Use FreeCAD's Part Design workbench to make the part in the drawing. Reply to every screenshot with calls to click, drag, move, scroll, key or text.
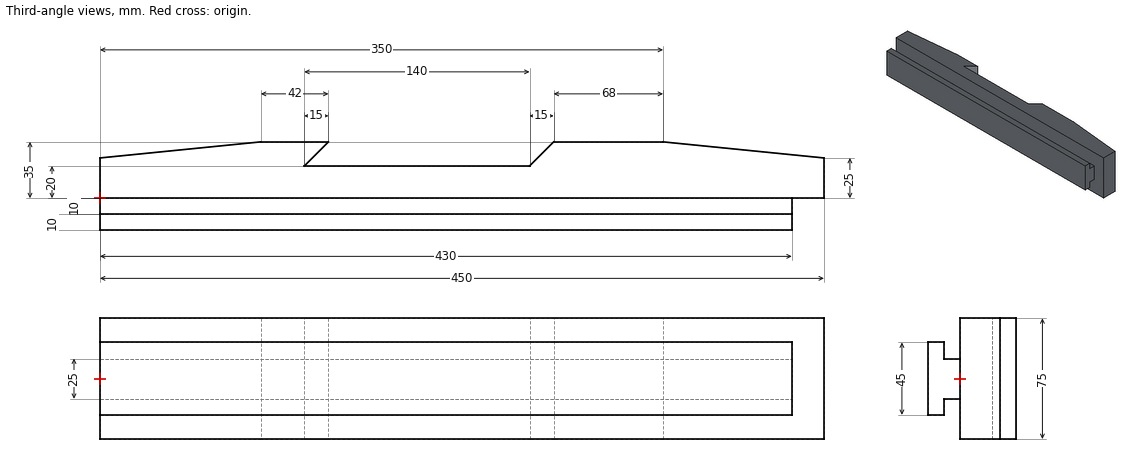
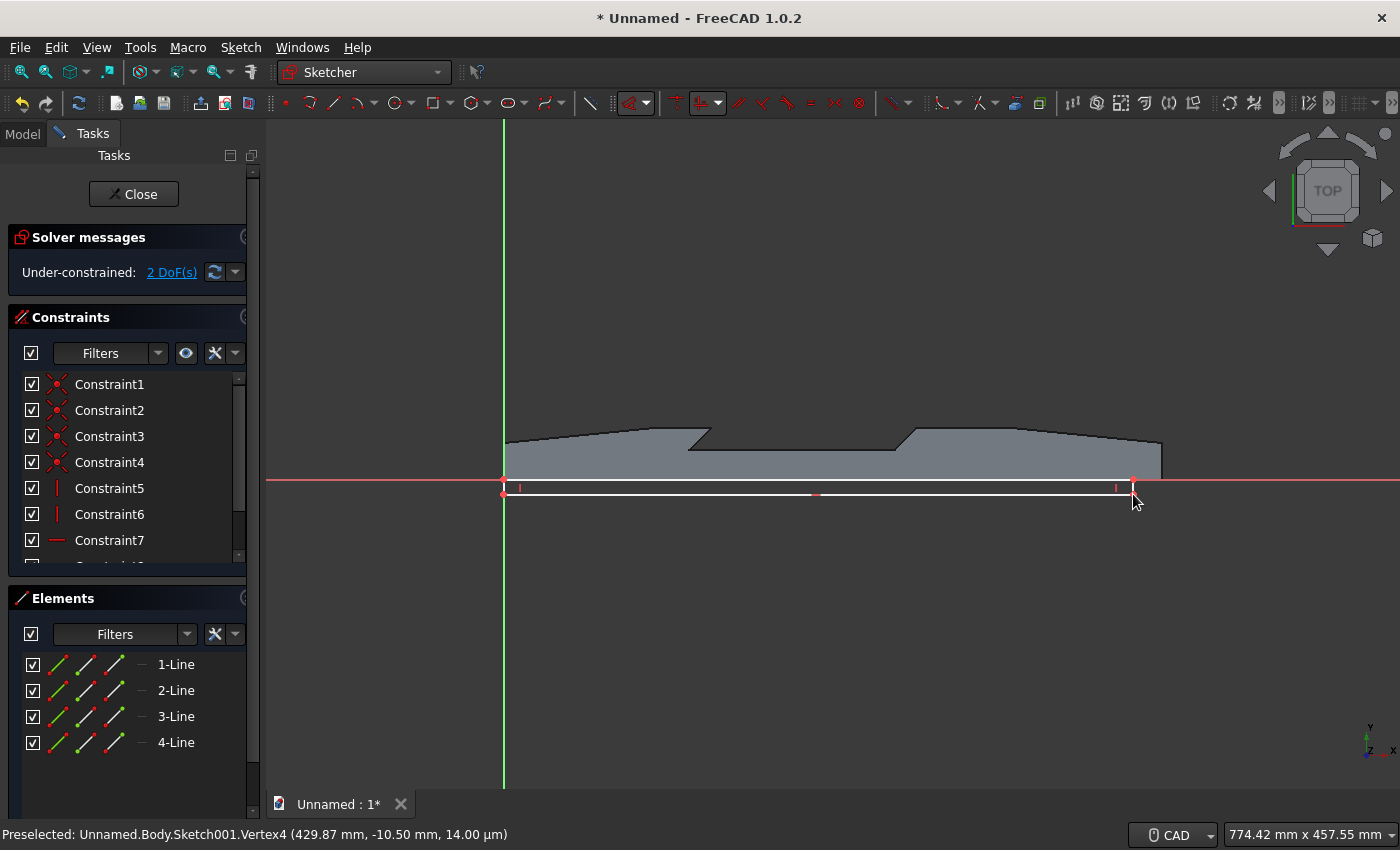
scroll(504, 487, up, 5)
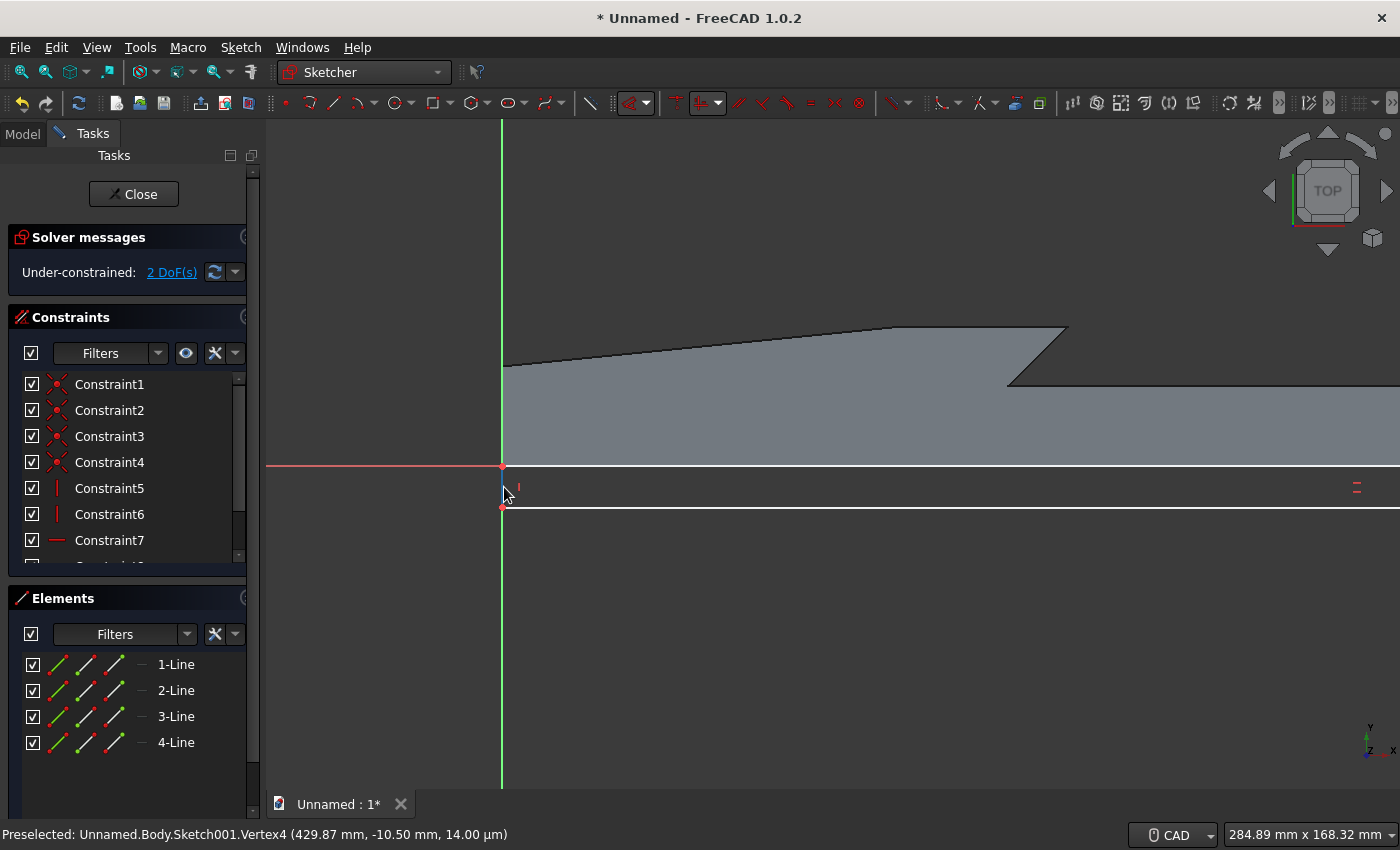
click(502, 487)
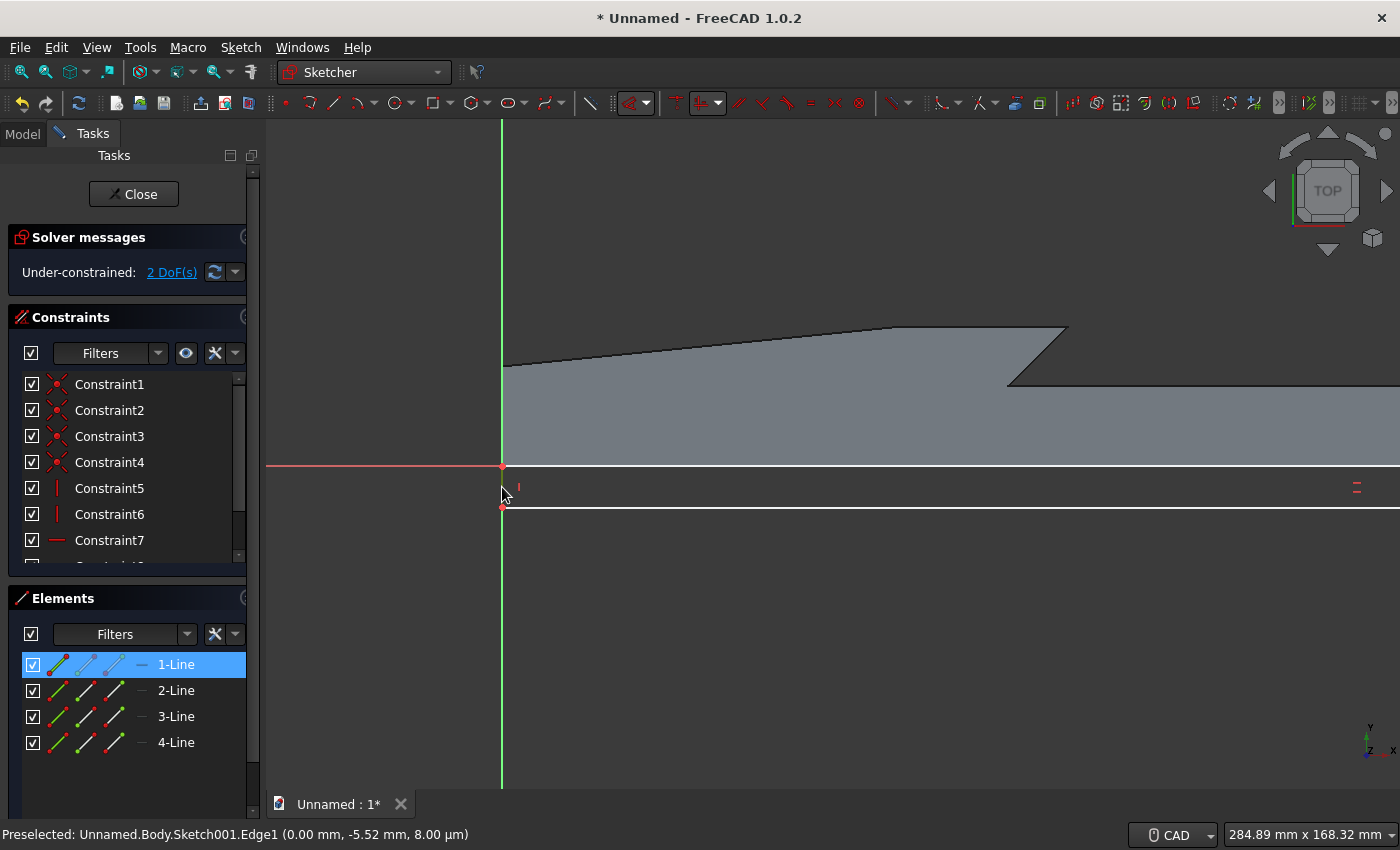
click(648, 104)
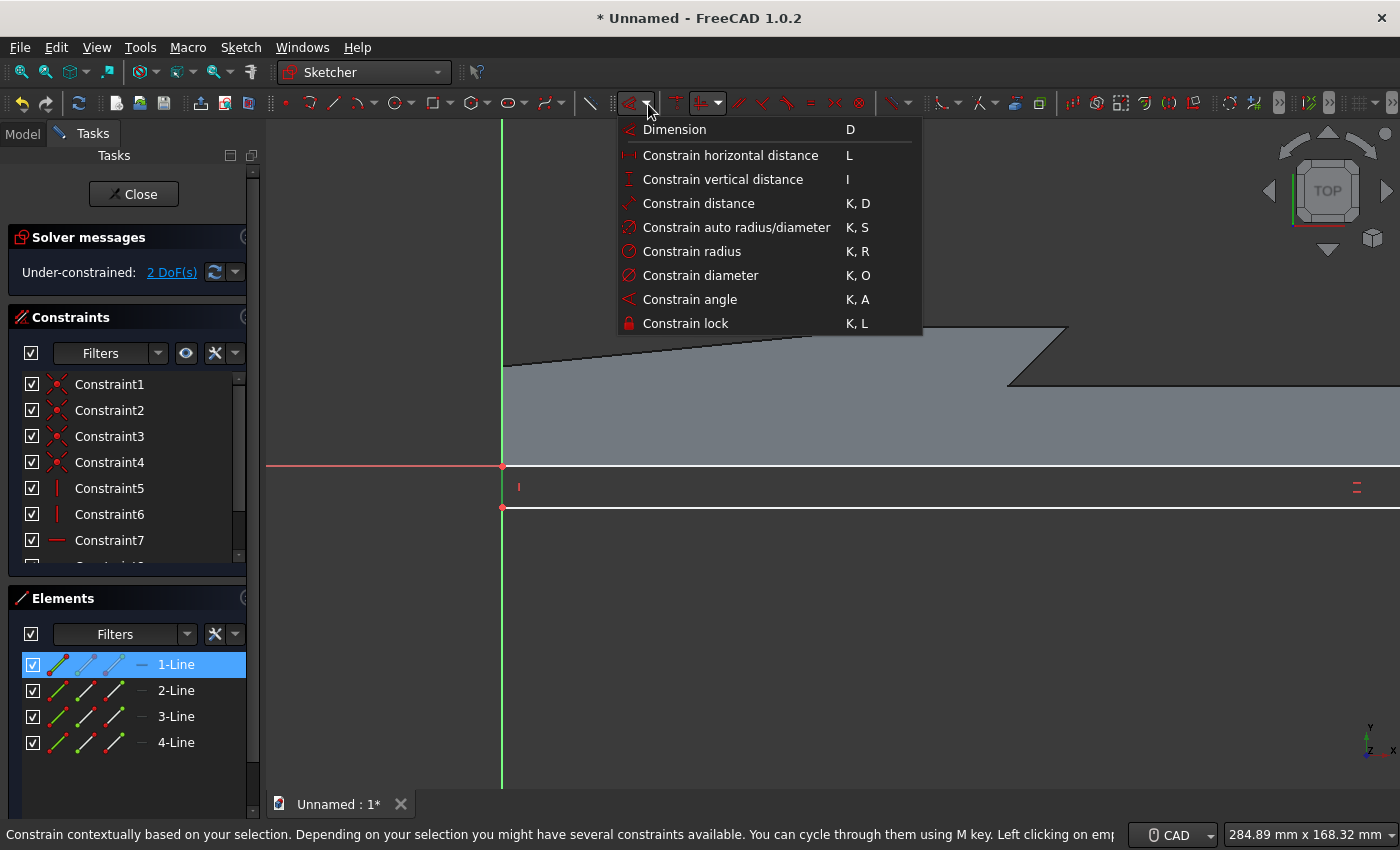
click(770, 179)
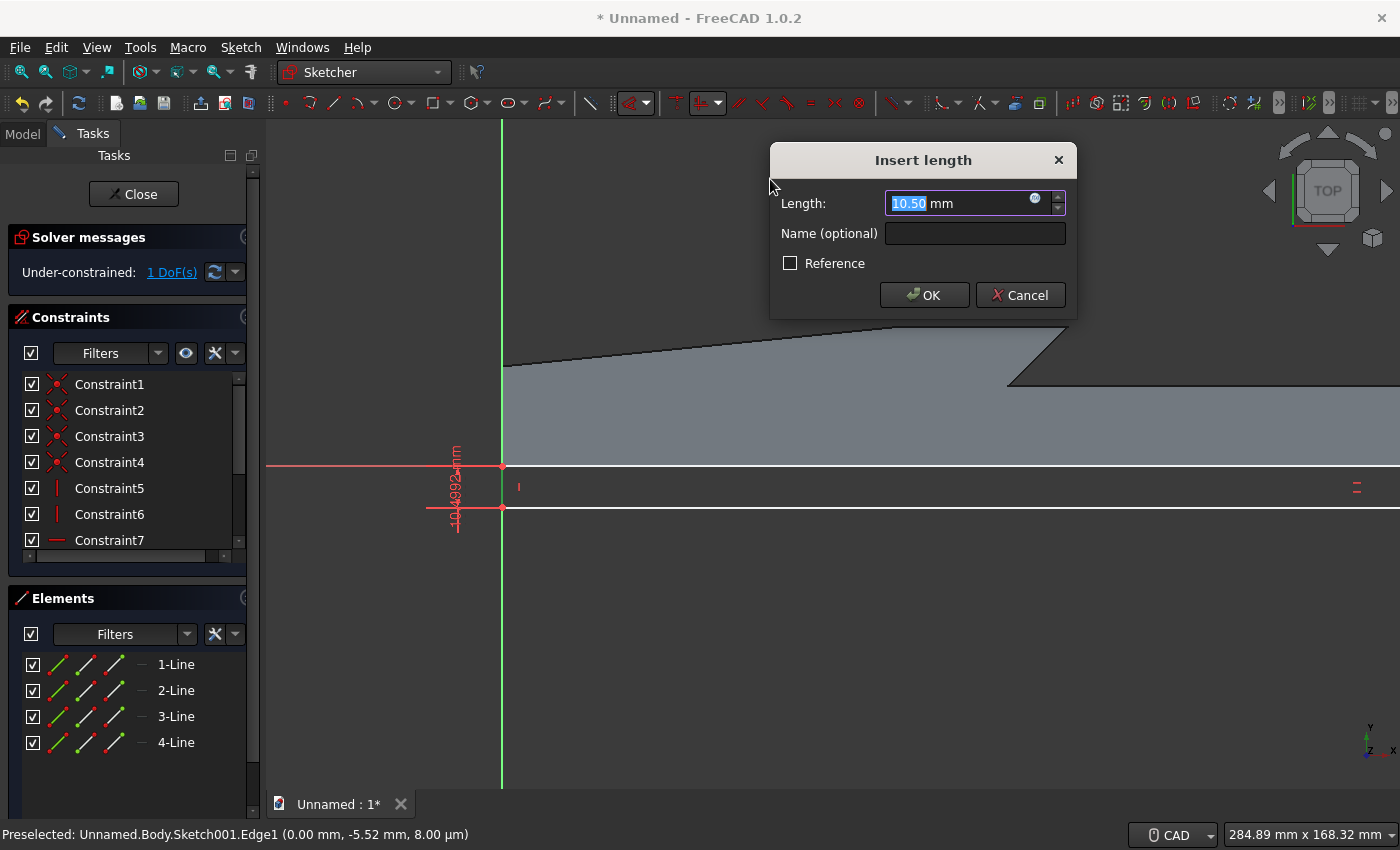
text(10)
key(Return)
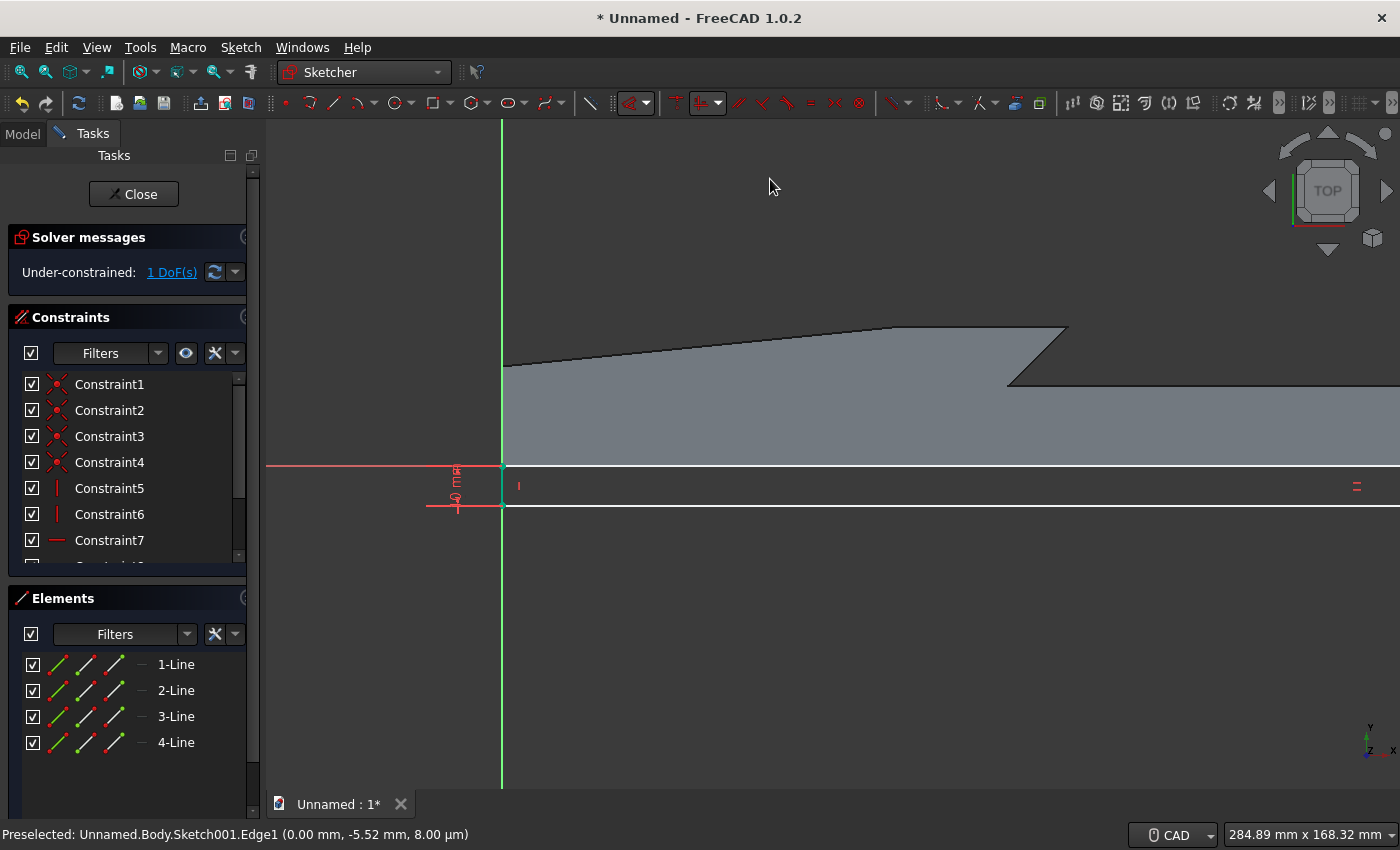
click(1016, 506)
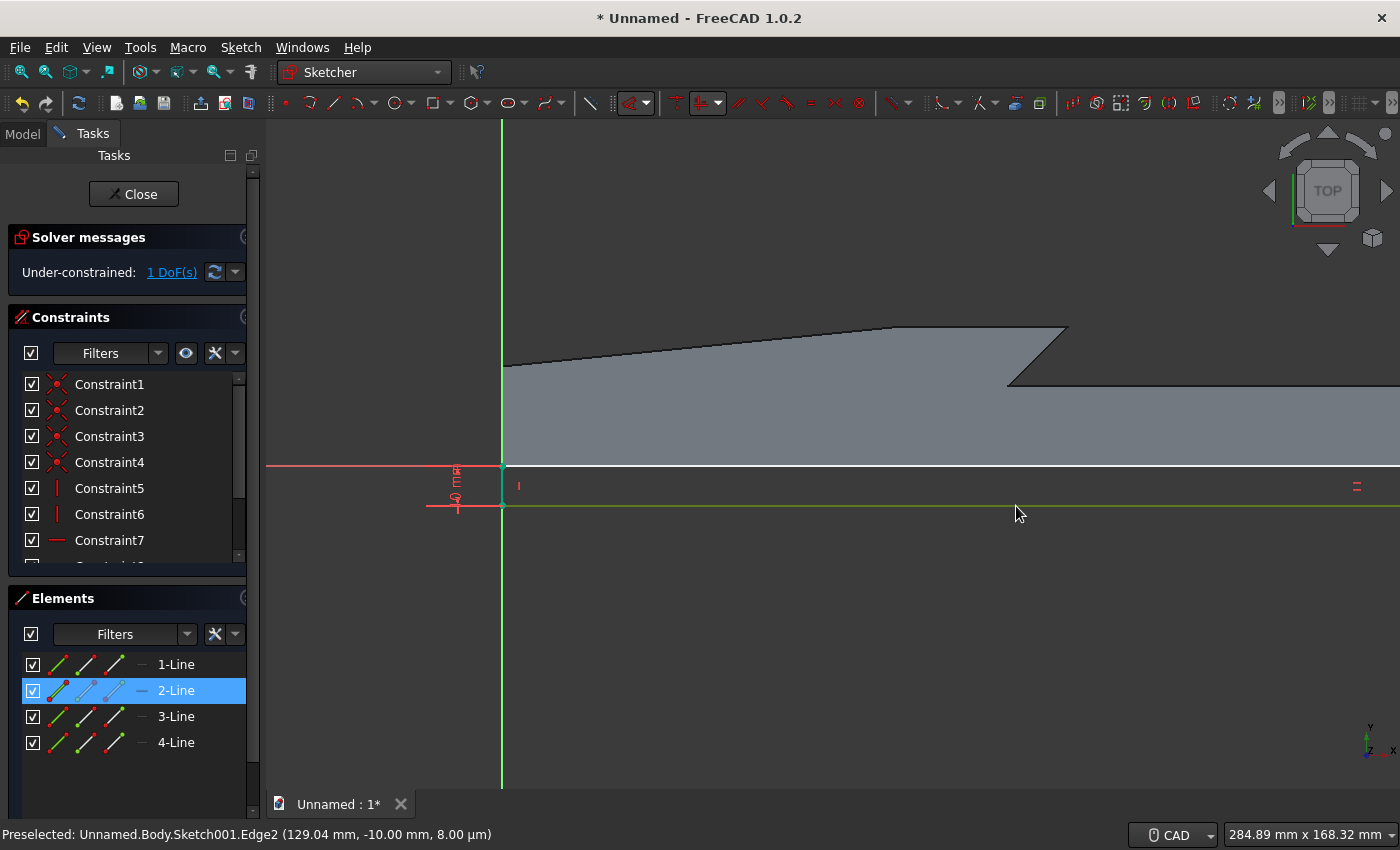
key(l)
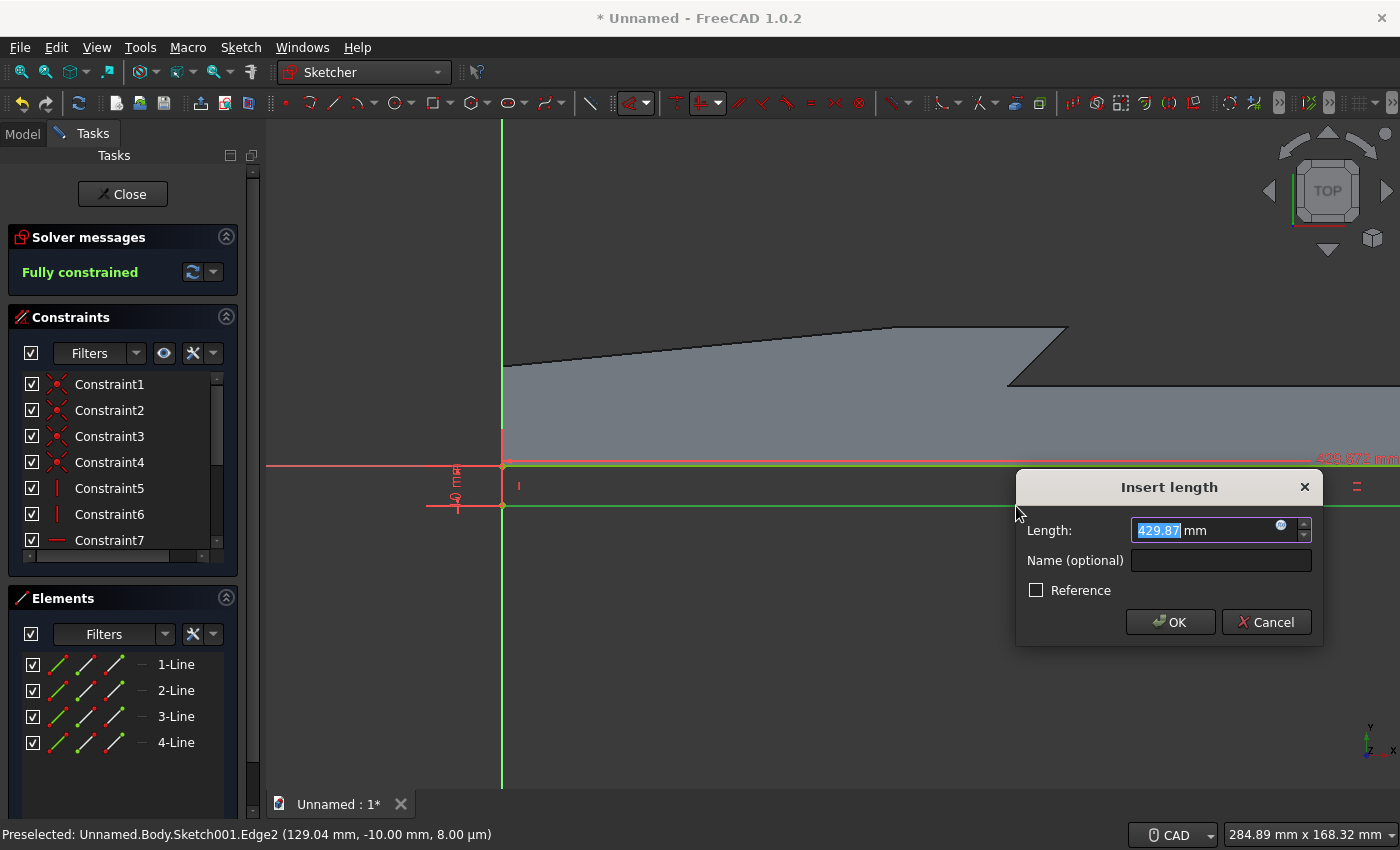
text(430)
key(Return)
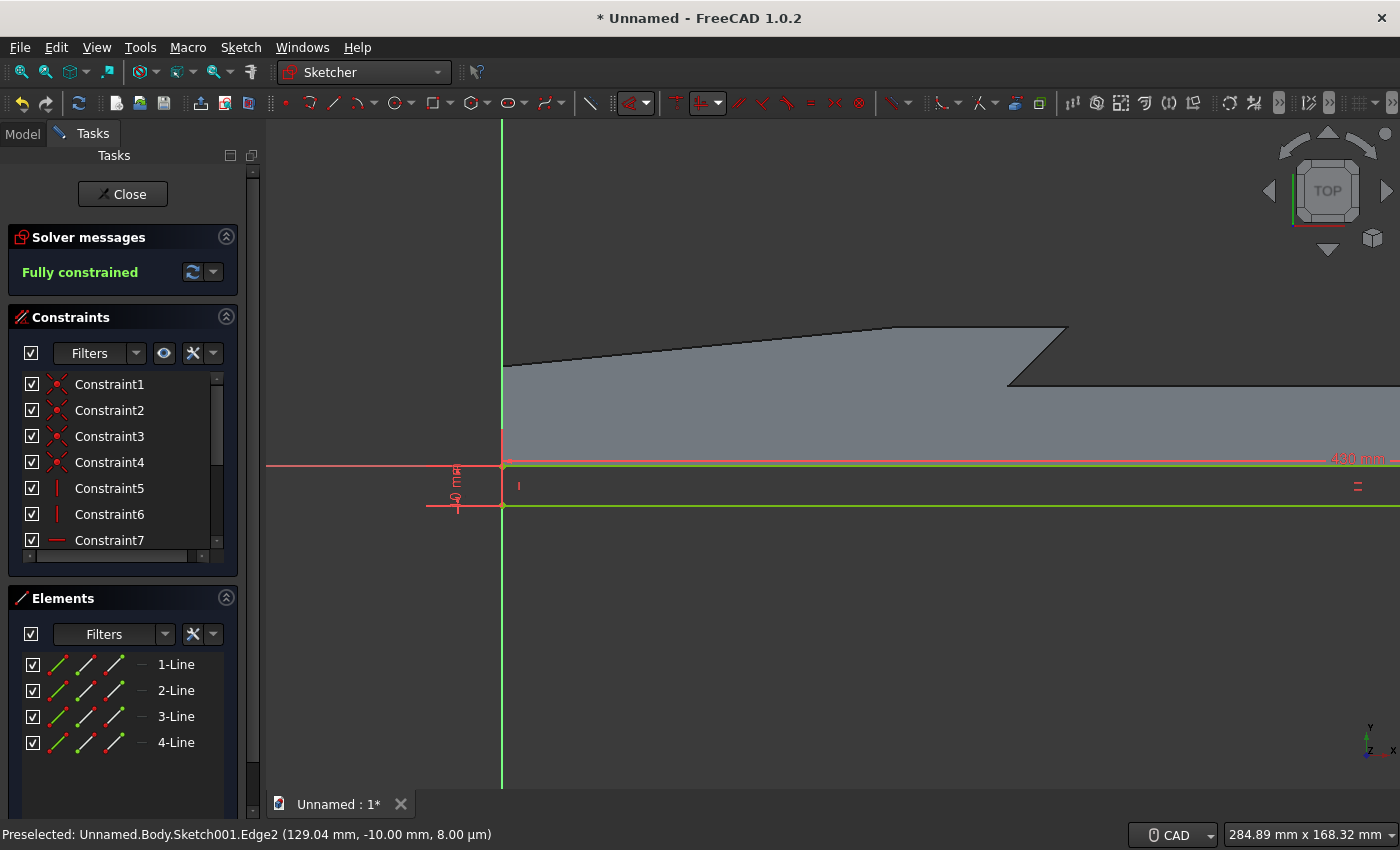
click(123, 194)